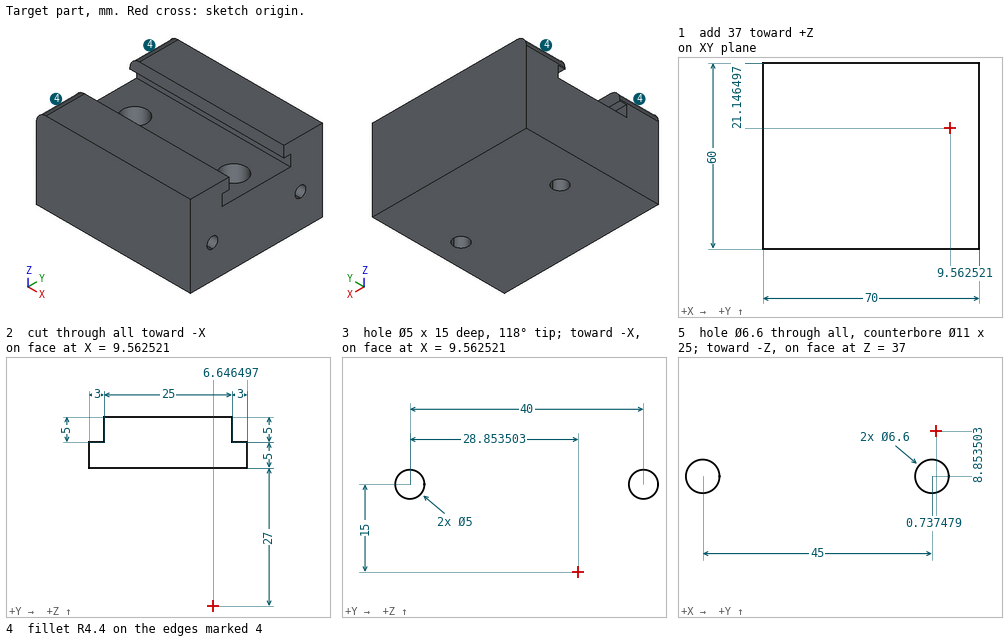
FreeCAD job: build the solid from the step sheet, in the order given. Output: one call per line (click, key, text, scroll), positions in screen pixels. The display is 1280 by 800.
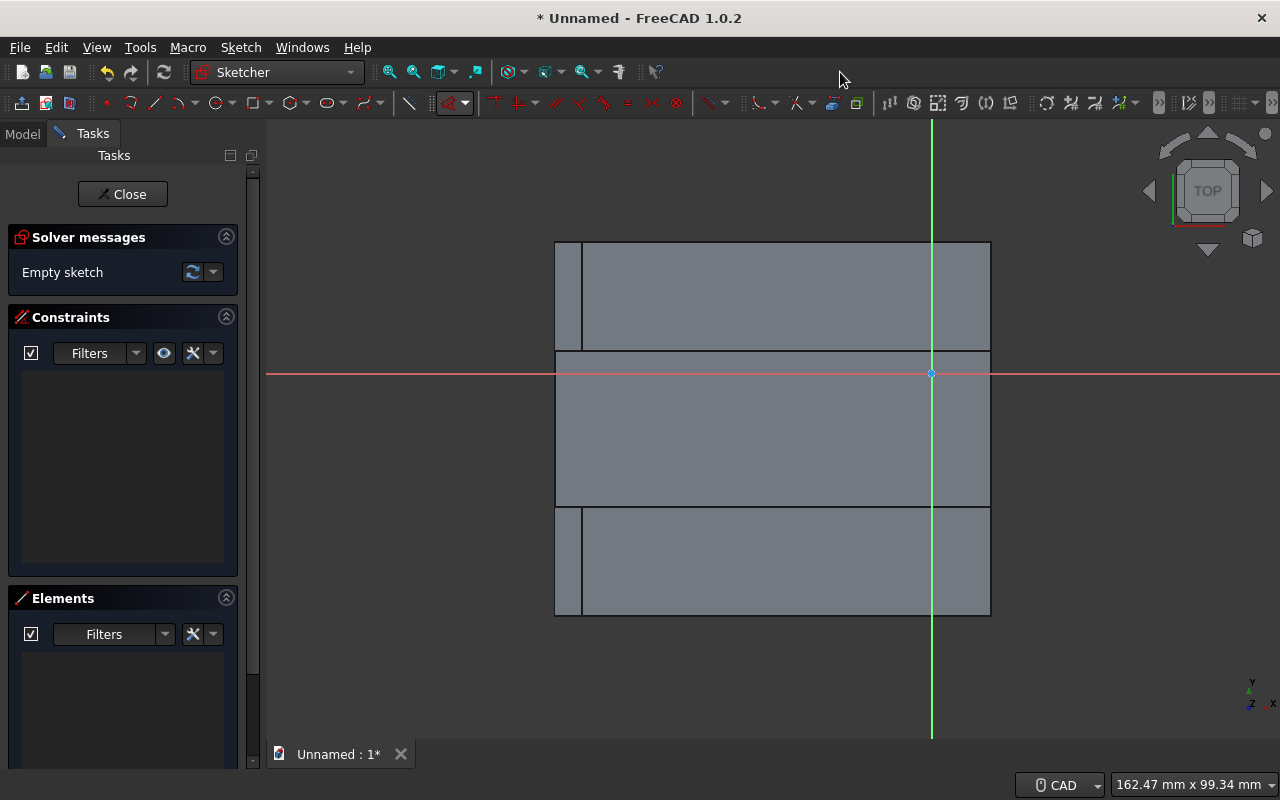
scroll(887, 391, up, 3)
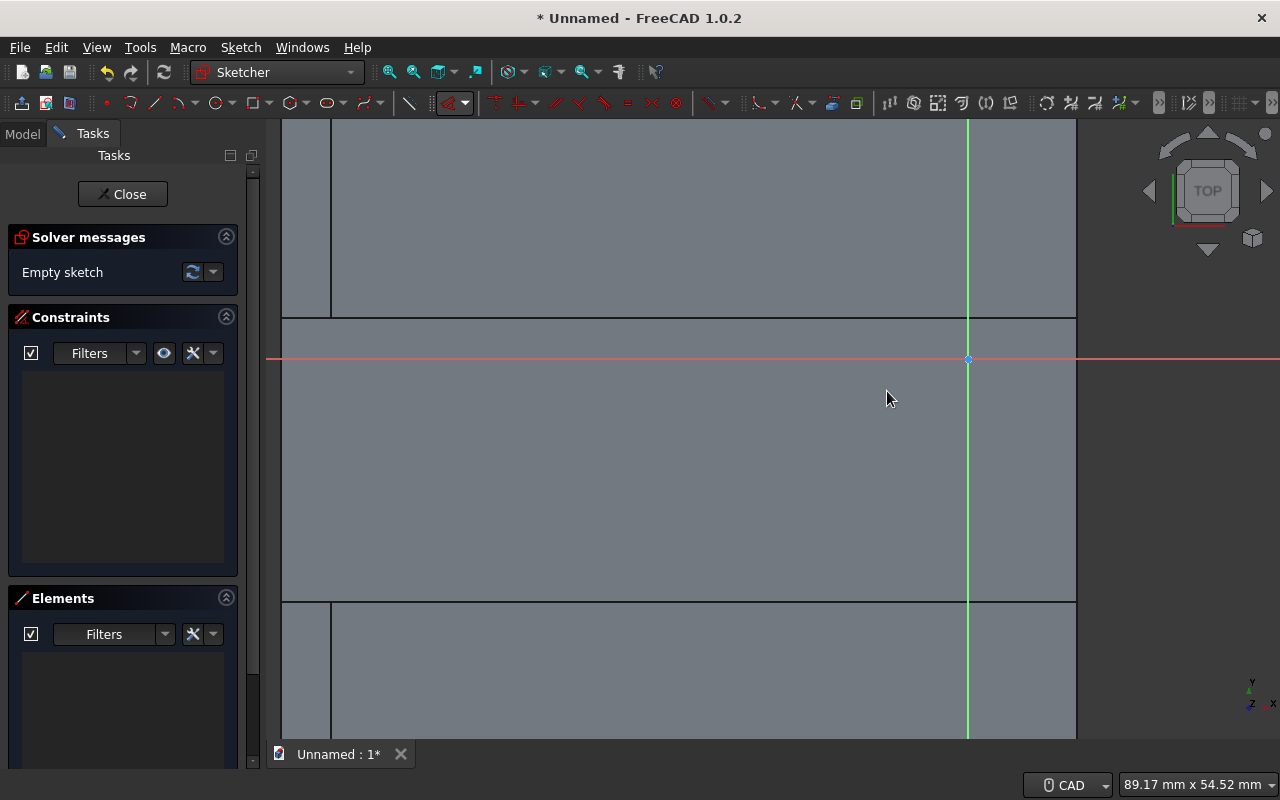
click(216, 104)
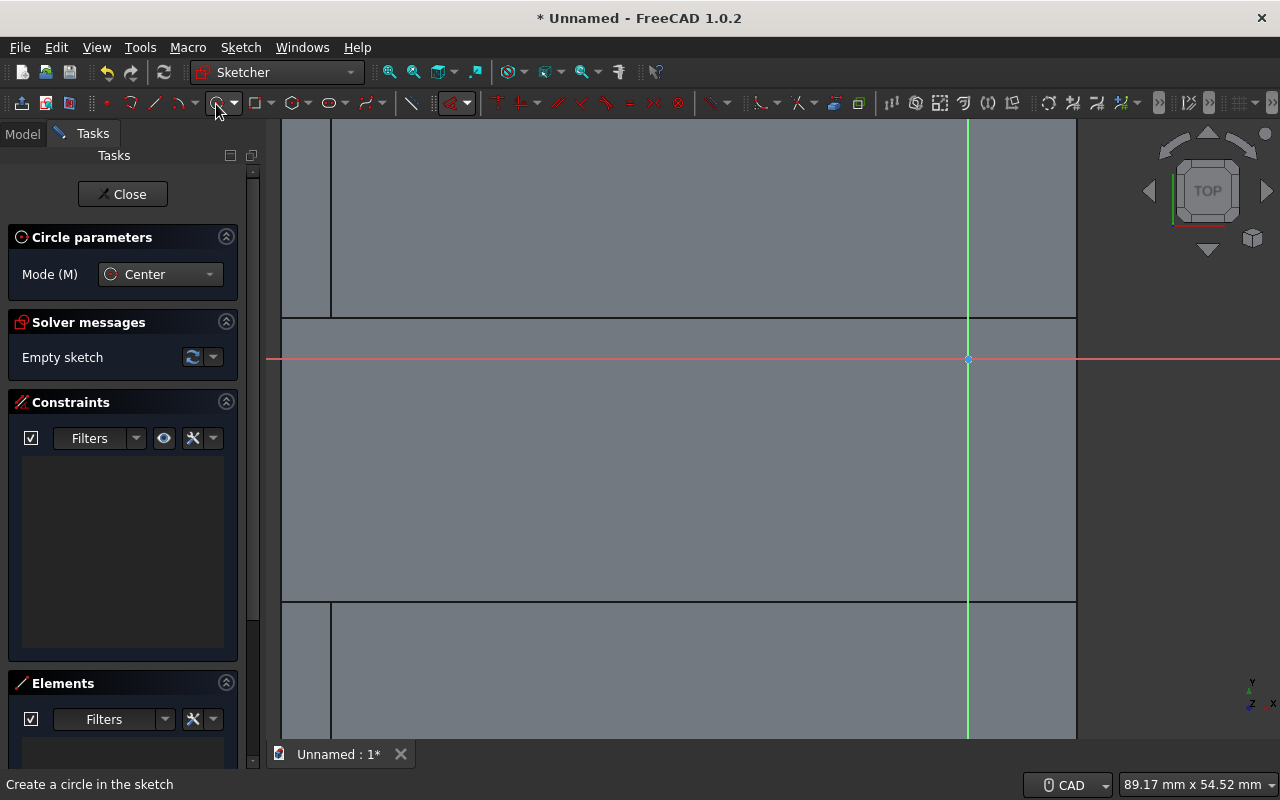
scroll(960, 460, up, 4)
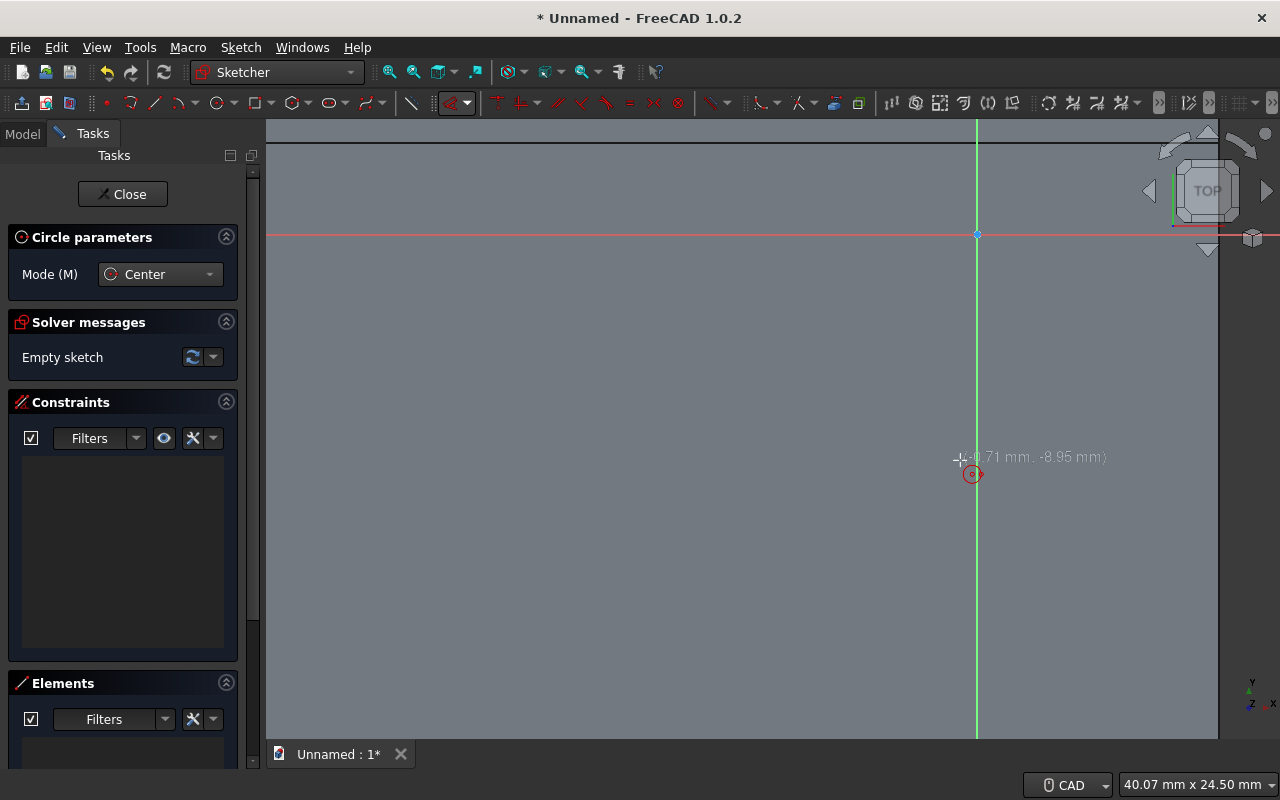
click(958, 459)
click(1017, 400)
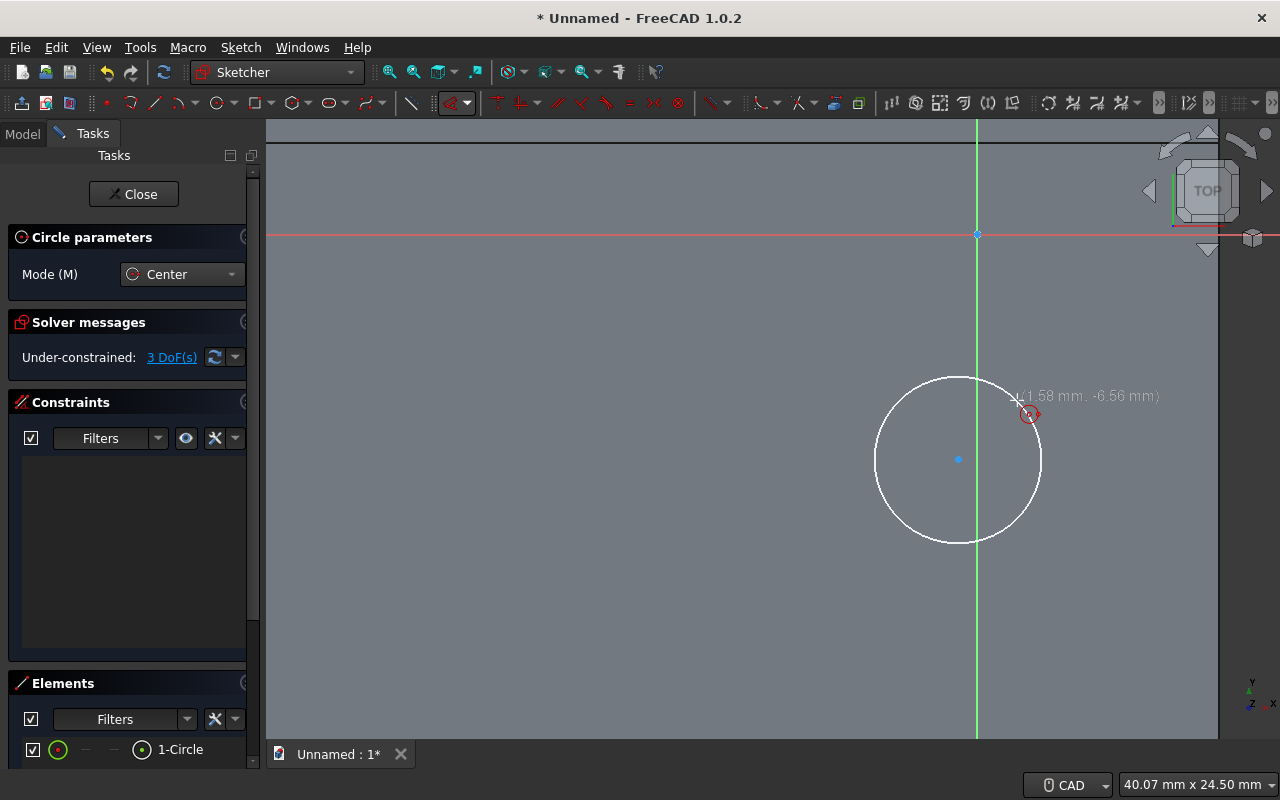
scroll(962, 462, down, 4)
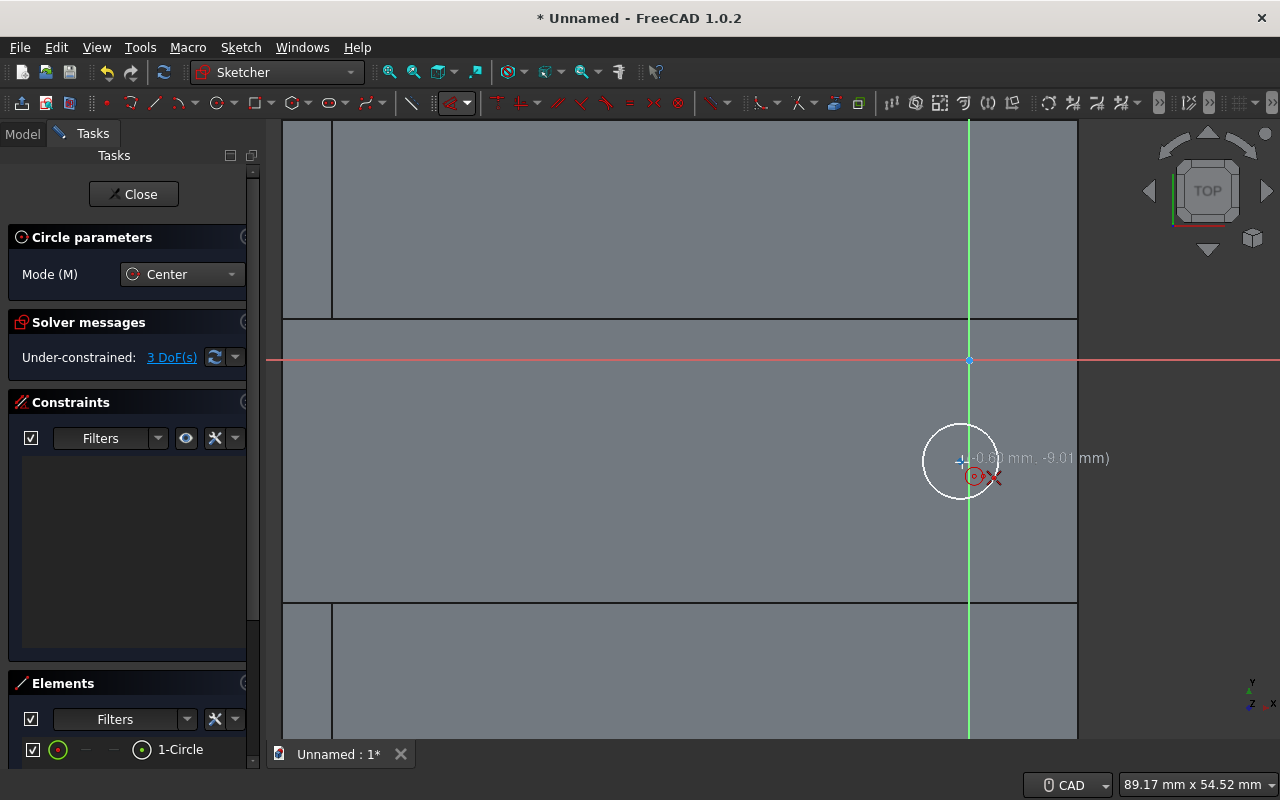
click(449, 461)
click(476, 434)
key(Escape)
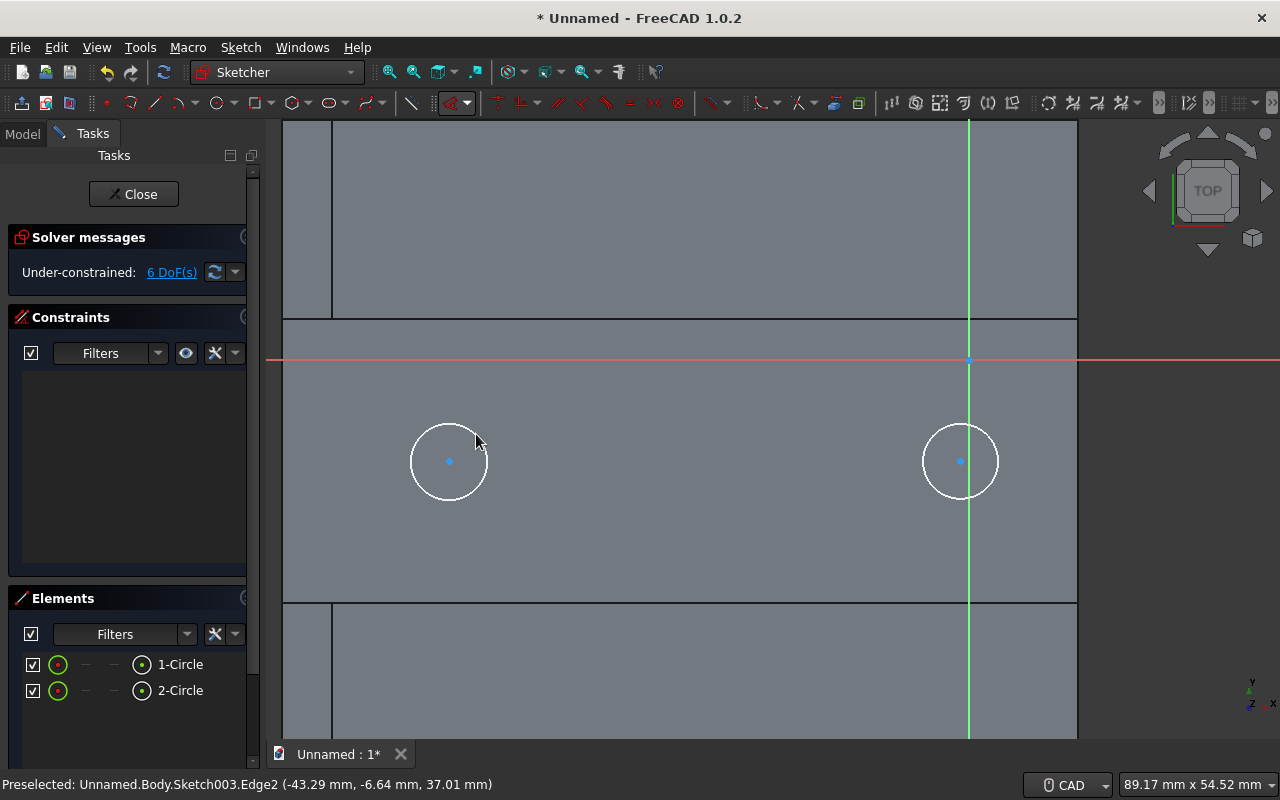
click(987, 435)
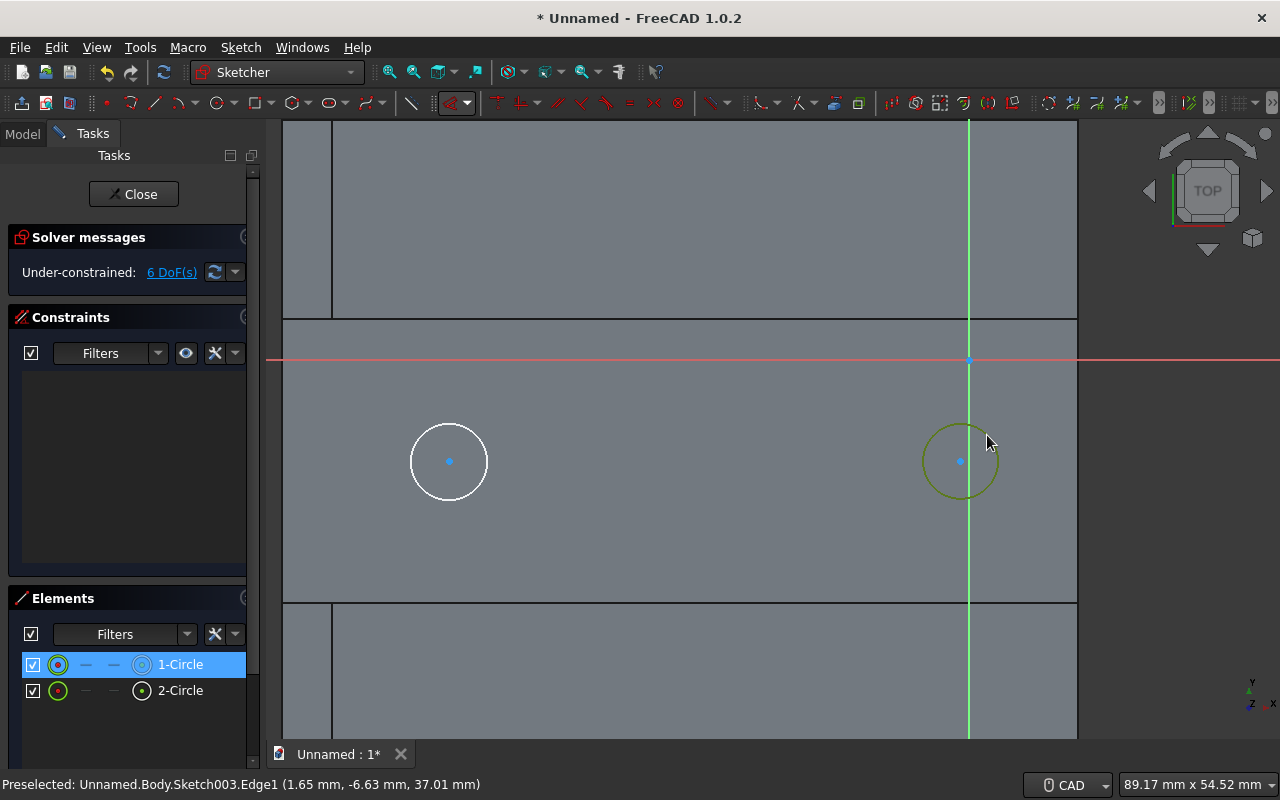
click(476, 435)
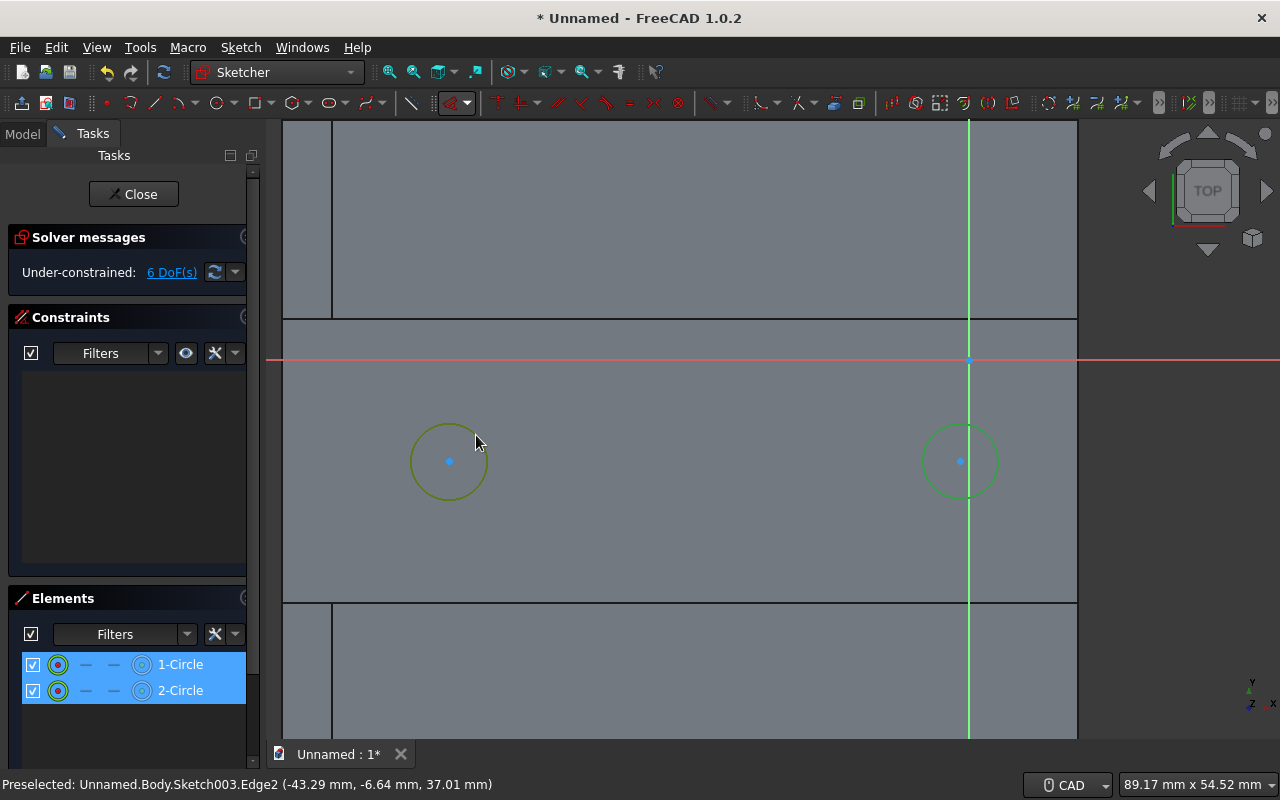
click(630, 104)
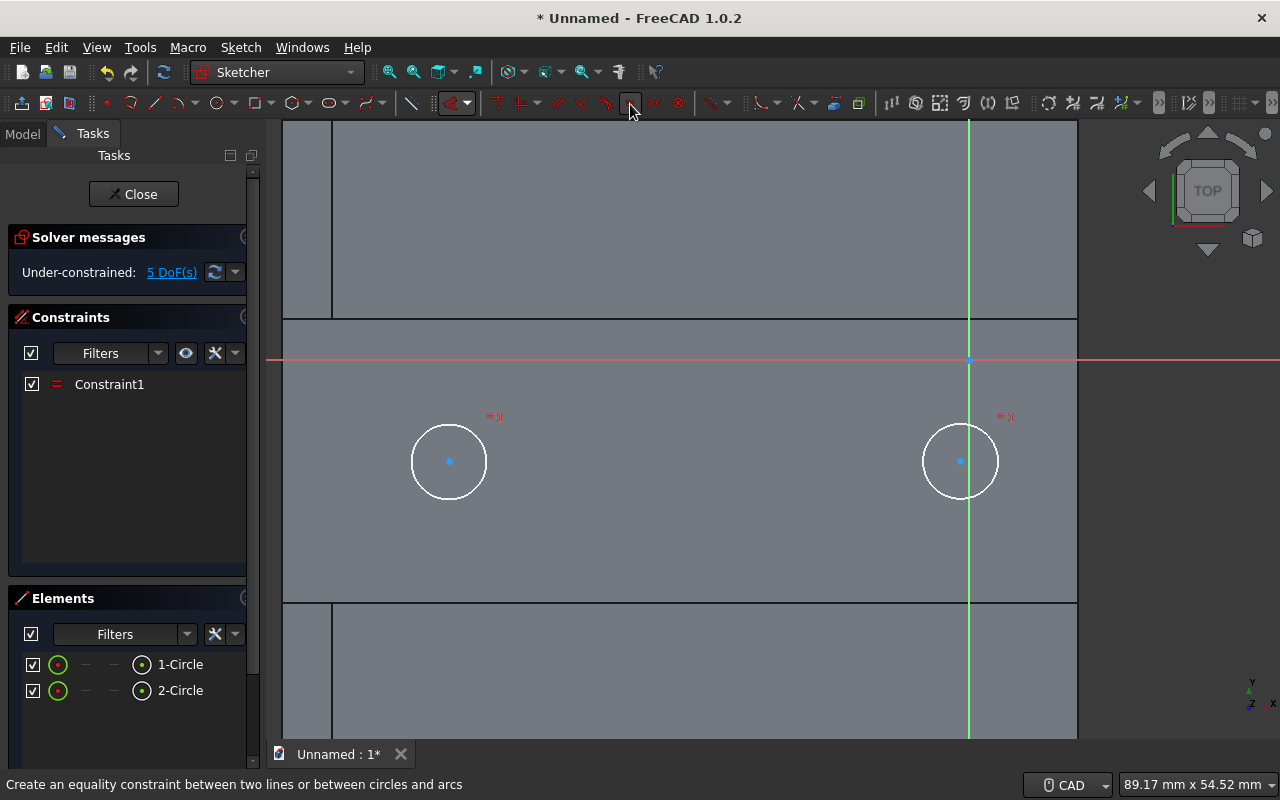
click(961, 461)